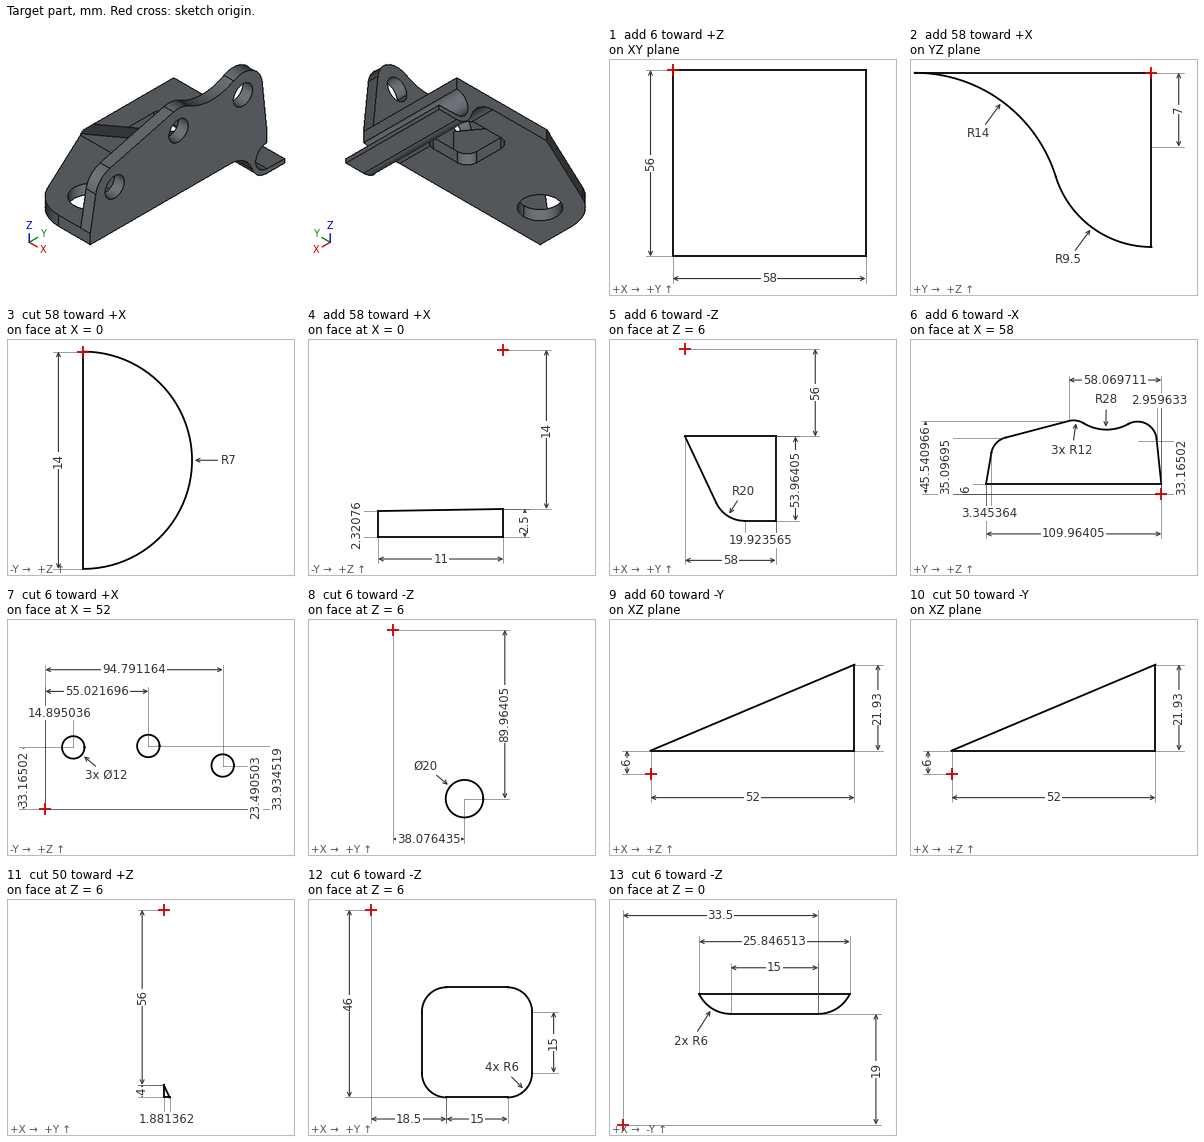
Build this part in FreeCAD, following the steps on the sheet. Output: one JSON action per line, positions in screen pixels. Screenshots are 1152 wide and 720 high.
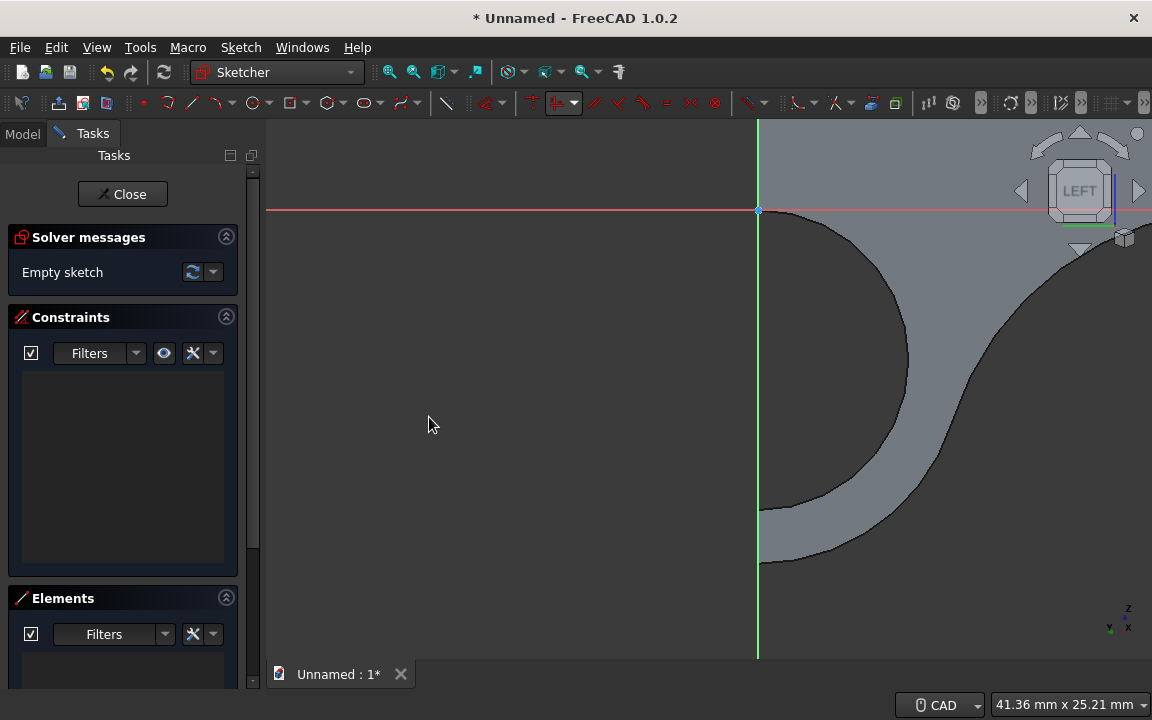
{"action": "left_click", "coordinate": [168, 104]}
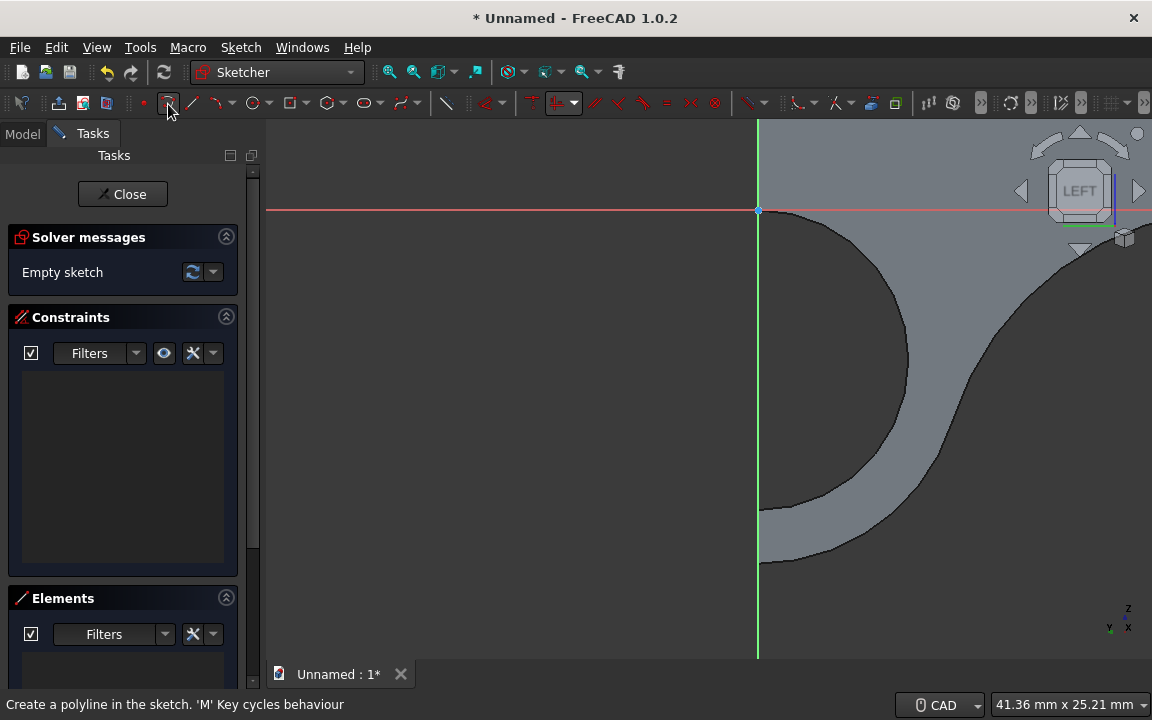
{"action": "left_click", "coordinate": [758, 510]}
{"action": "left_click", "coordinate": [523, 522]}
{"action": "left_click", "coordinate": [523, 564]}
{"action": "left_click", "coordinate": [749, 564]}
{"action": "left_click", "coordinate": [758, 511]}
{"action": "key", "text": "Escape"}
{"action": "key", "text": "Escape"}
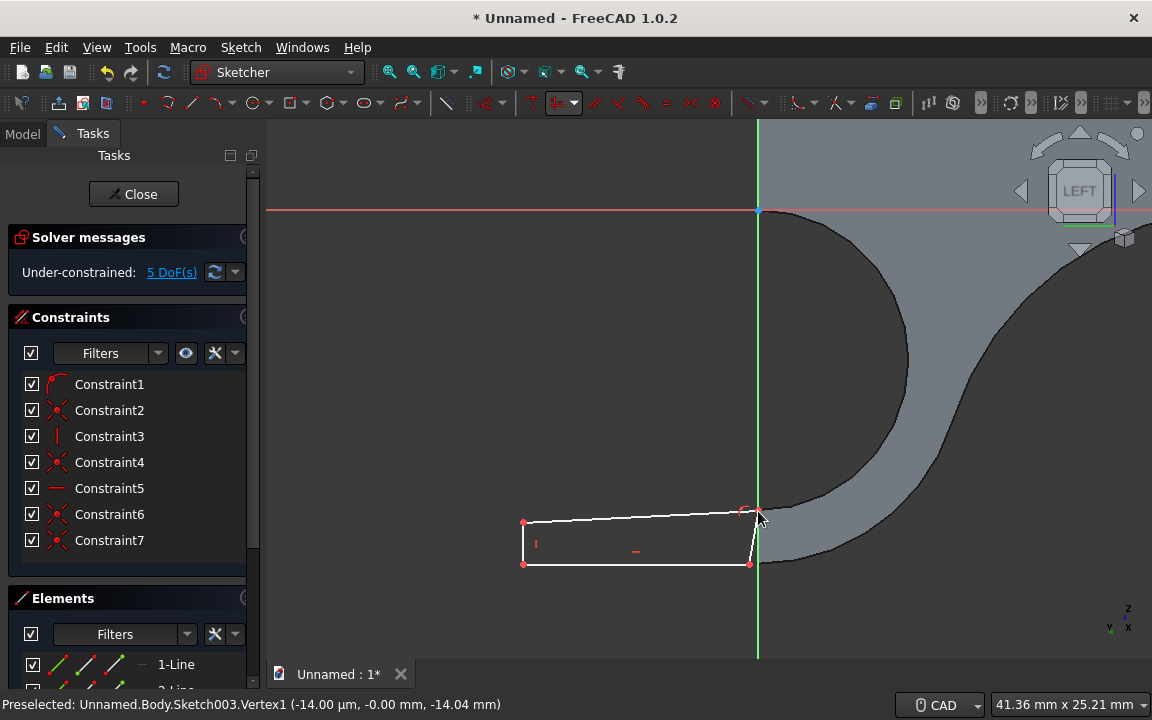
{"action": "left_click", "coordinate": [756, 527]}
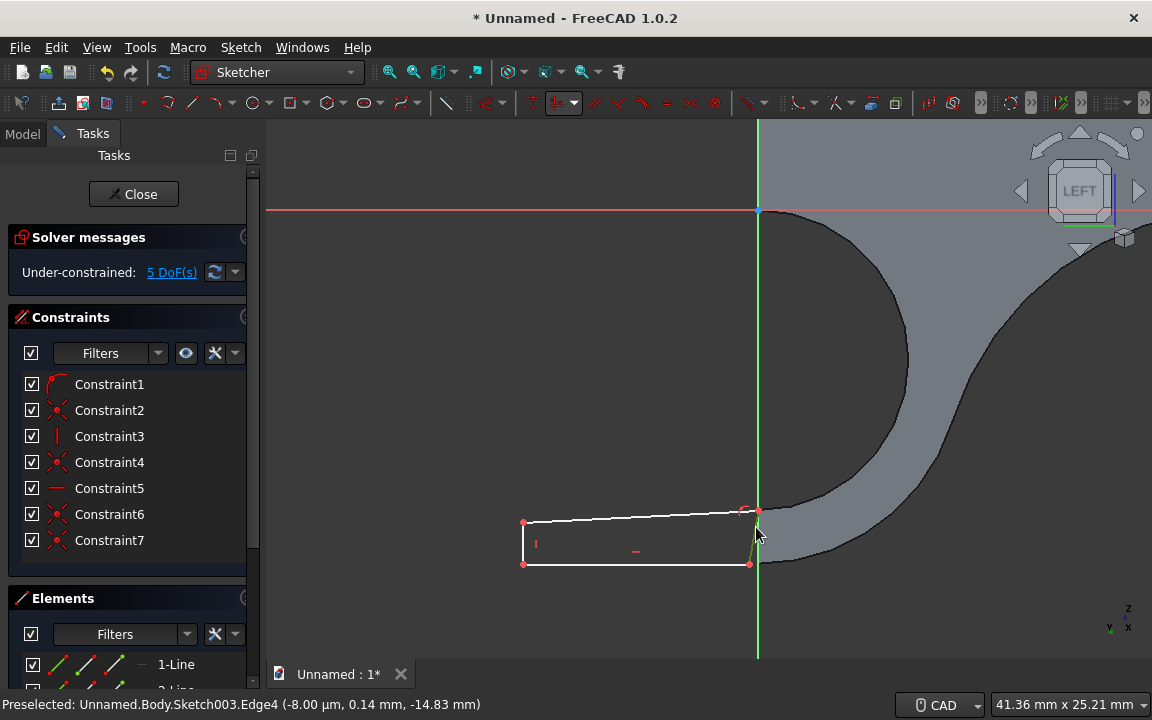
{"action": "left_click", "coordinate": [576, 104]}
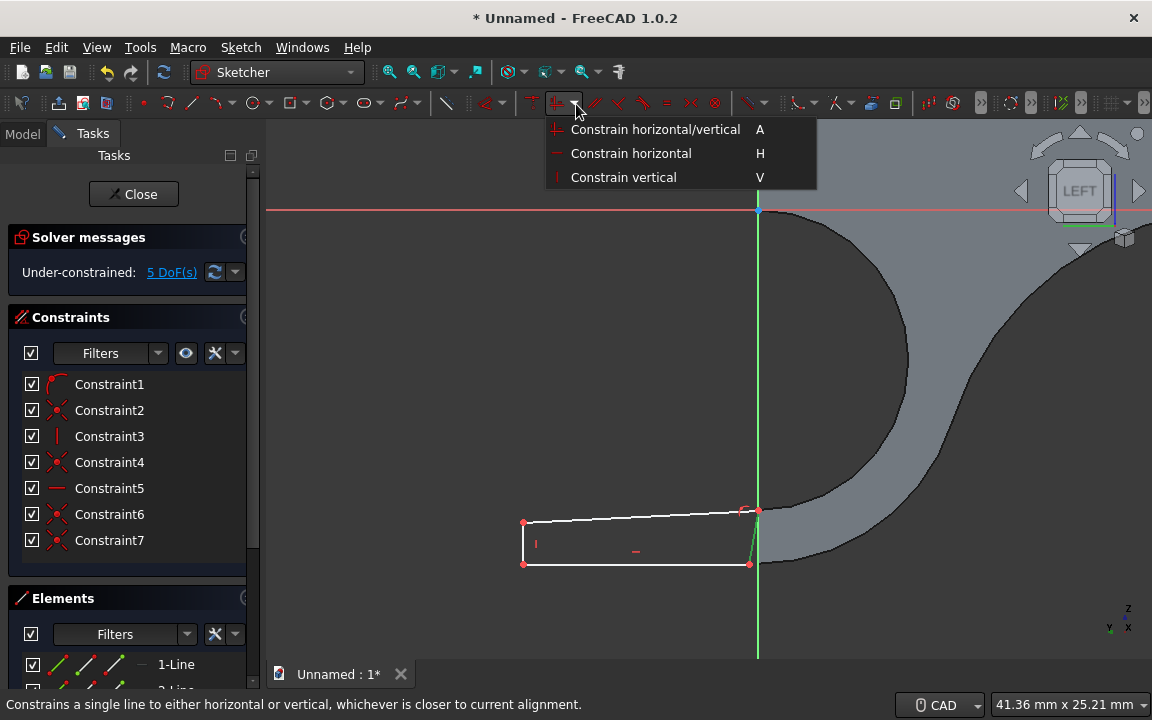
{"action": "left_click", "coordinate": [681, 177]}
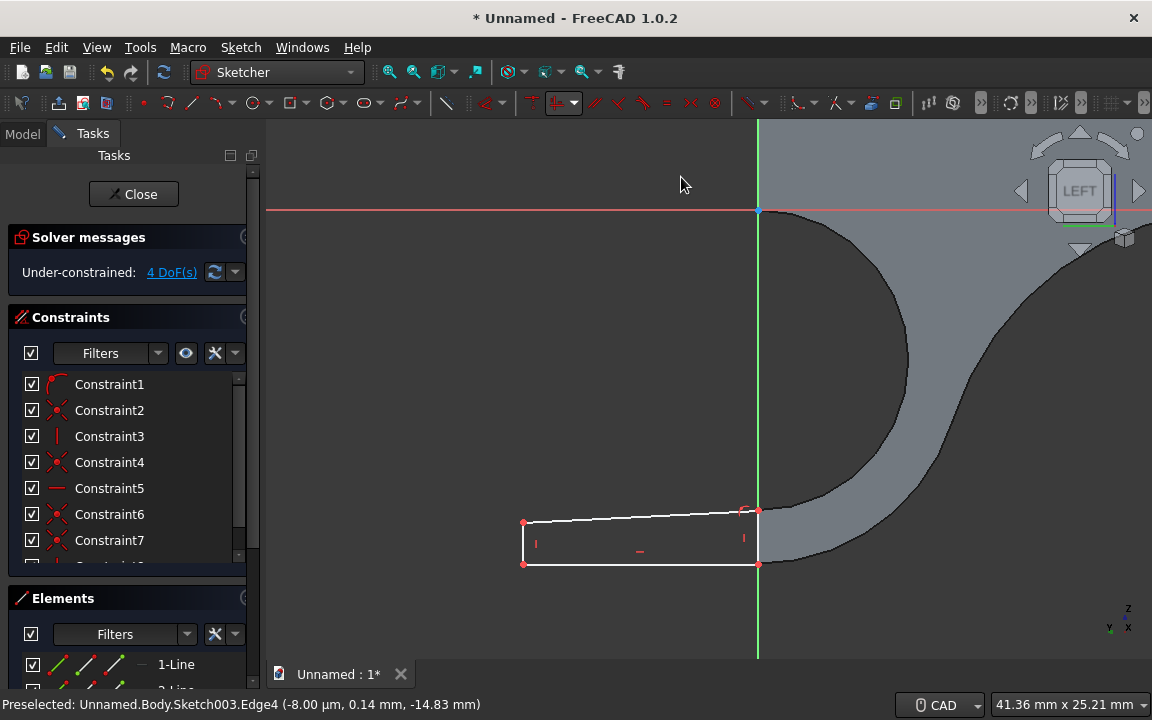
{"action": "left_click", "coordinate": [486, 104]}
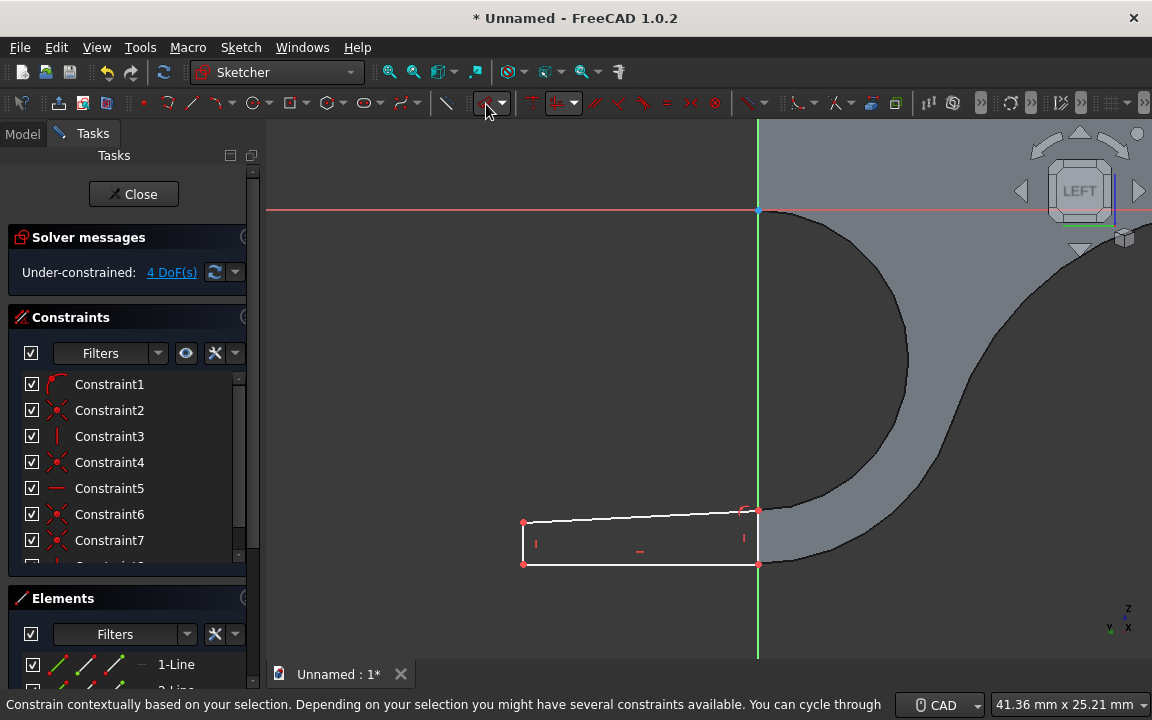
{"action": "left_click", "coordinate": [594, 565]}
{"action": "left_click", "coordinate": [641, 599]}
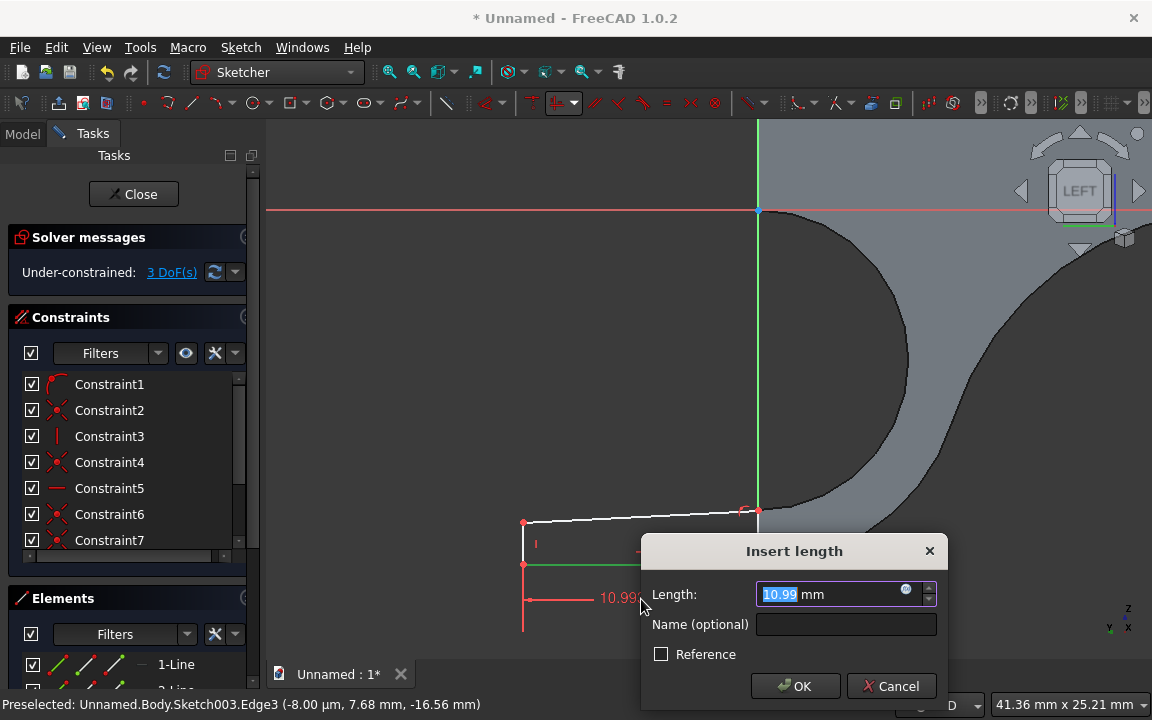
{"action": "type", "text": "11"}
{"action": "key", "text": "Return"}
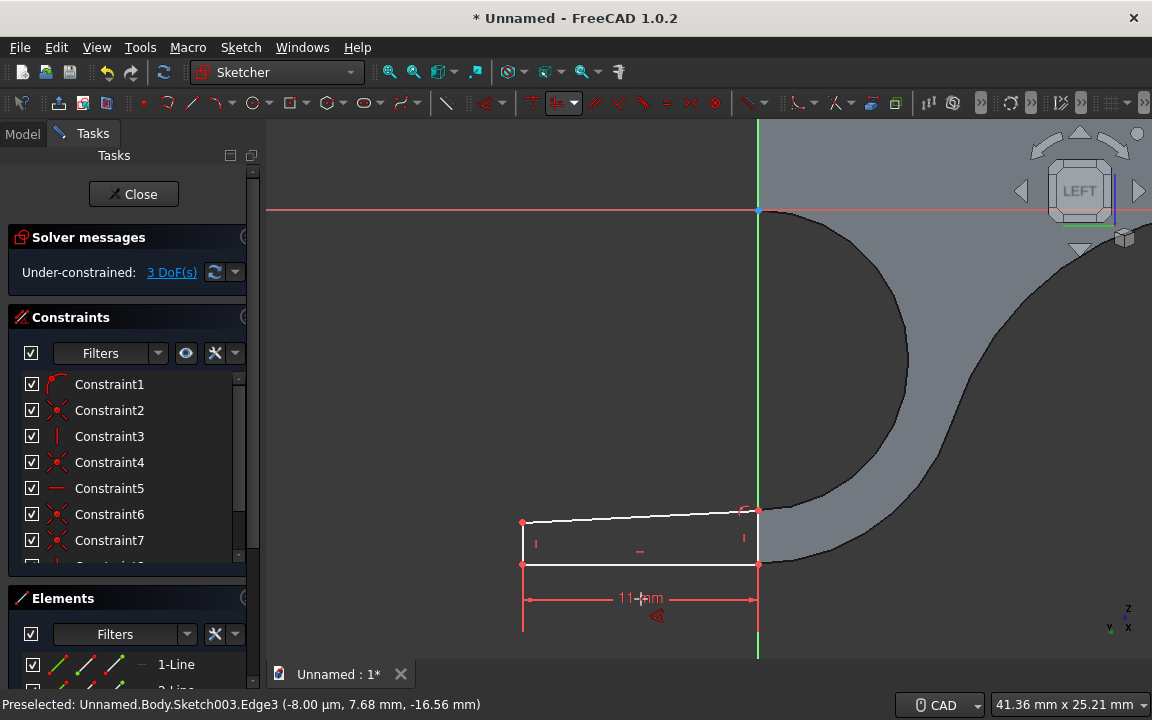
{"action": "left_click", "coordinate": [758, 549]}
{"action": "left_click", "coordinate": [792, 538]}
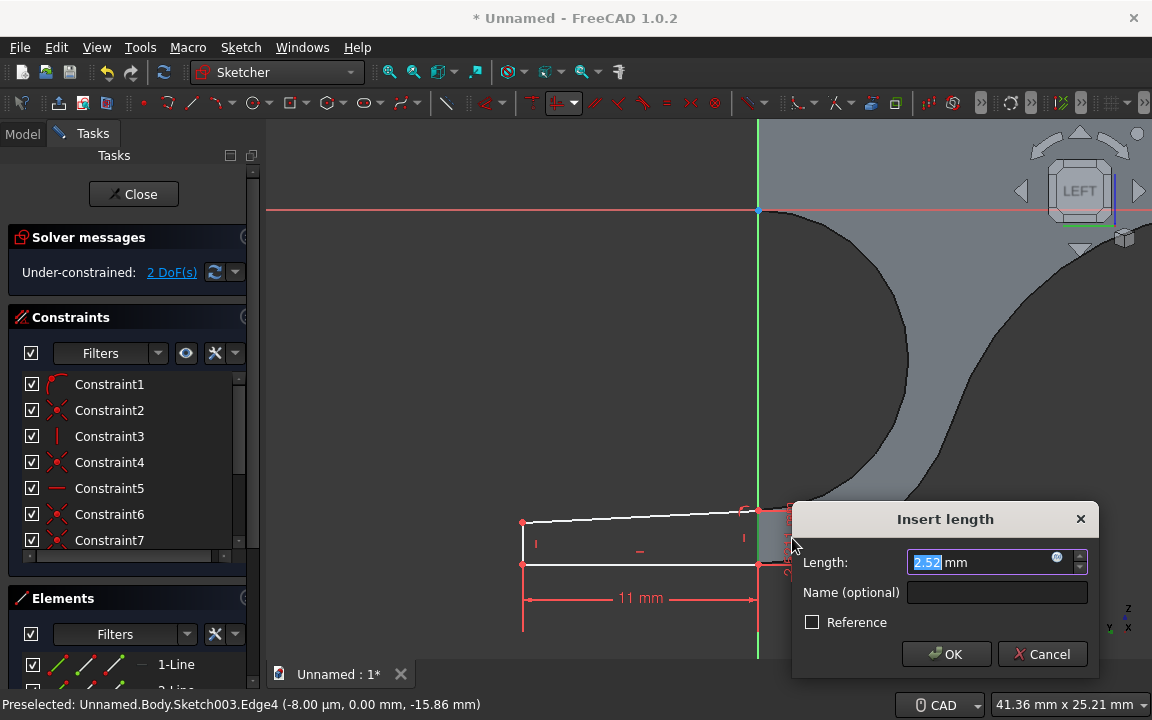
{"action": "type", "text": "2.5"}
{"action": "key", "text": "Return"}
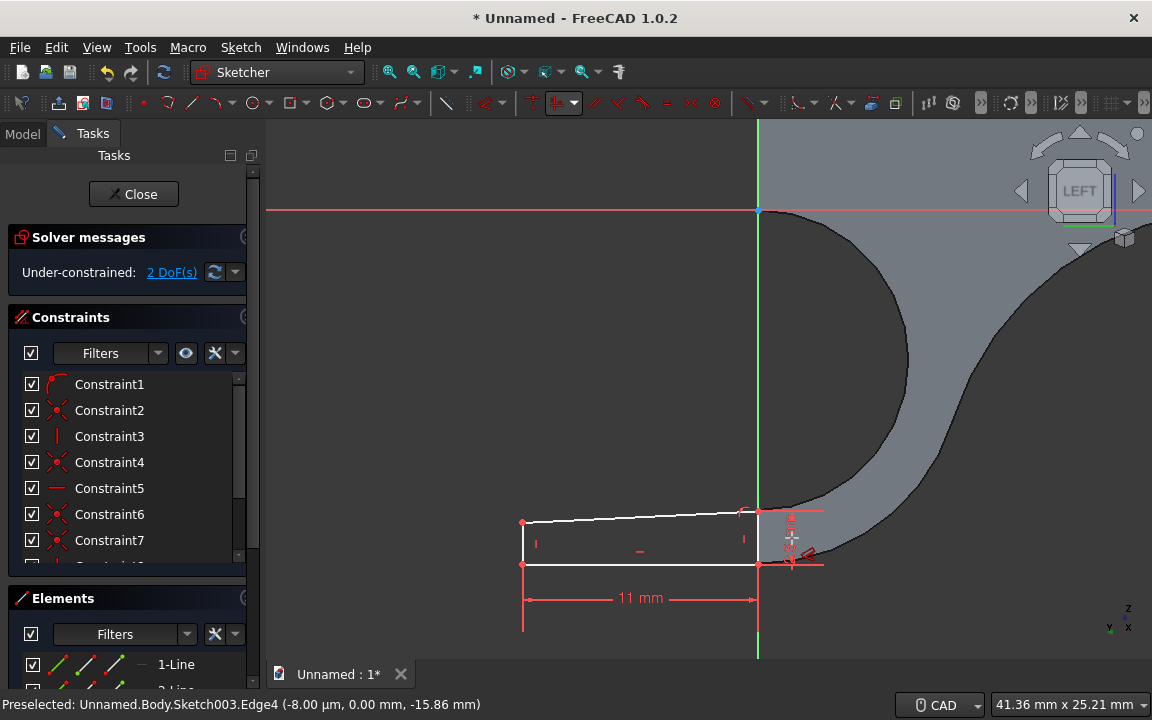
{"action": "left_click", "coordinate": [758, 511]}
{"action": "left_click", "coordinate": [792, 361]}